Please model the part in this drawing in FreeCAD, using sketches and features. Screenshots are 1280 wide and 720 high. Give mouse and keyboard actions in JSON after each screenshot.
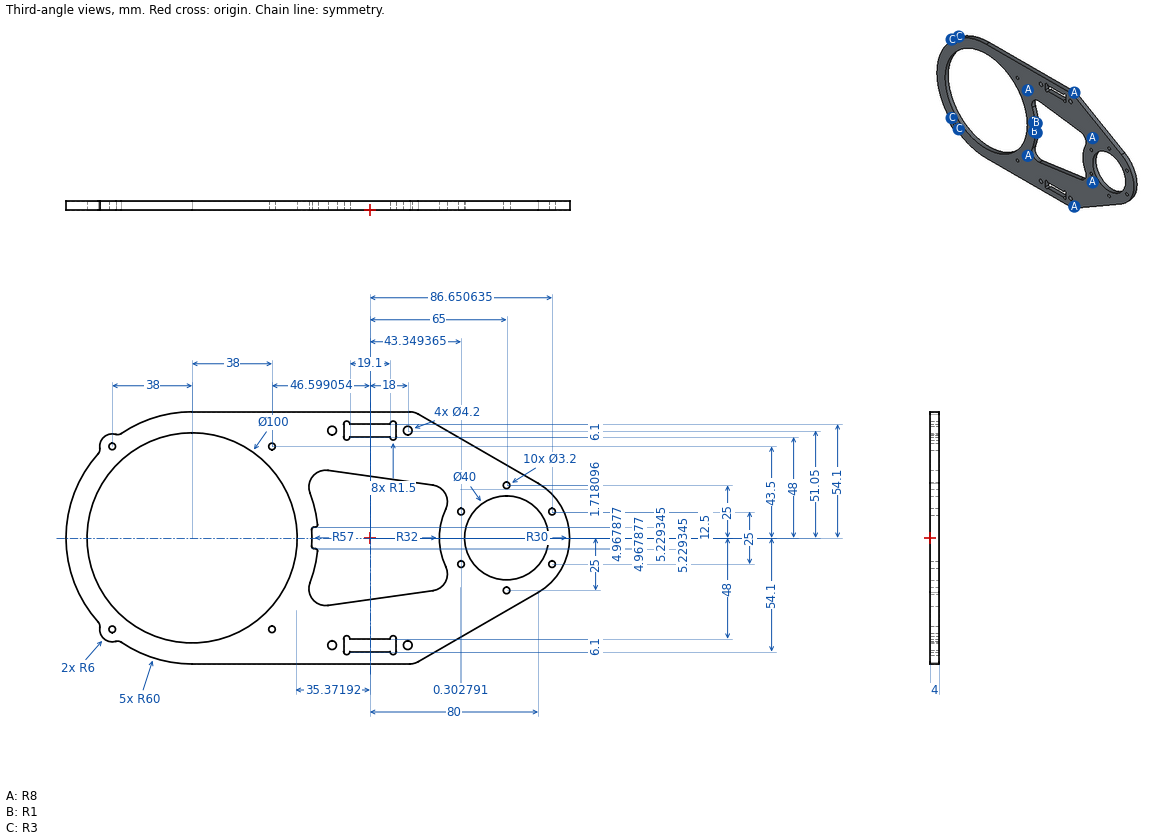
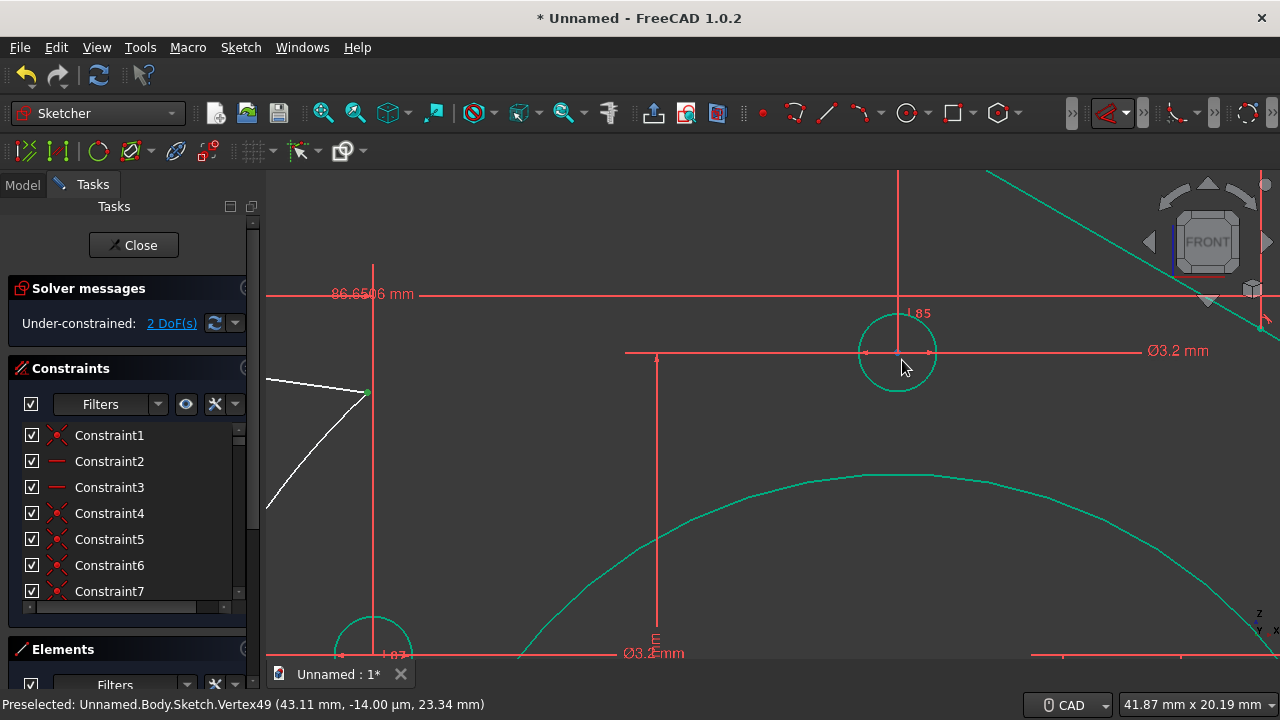
{"action": "left_click", "coordinate": [898, 353]}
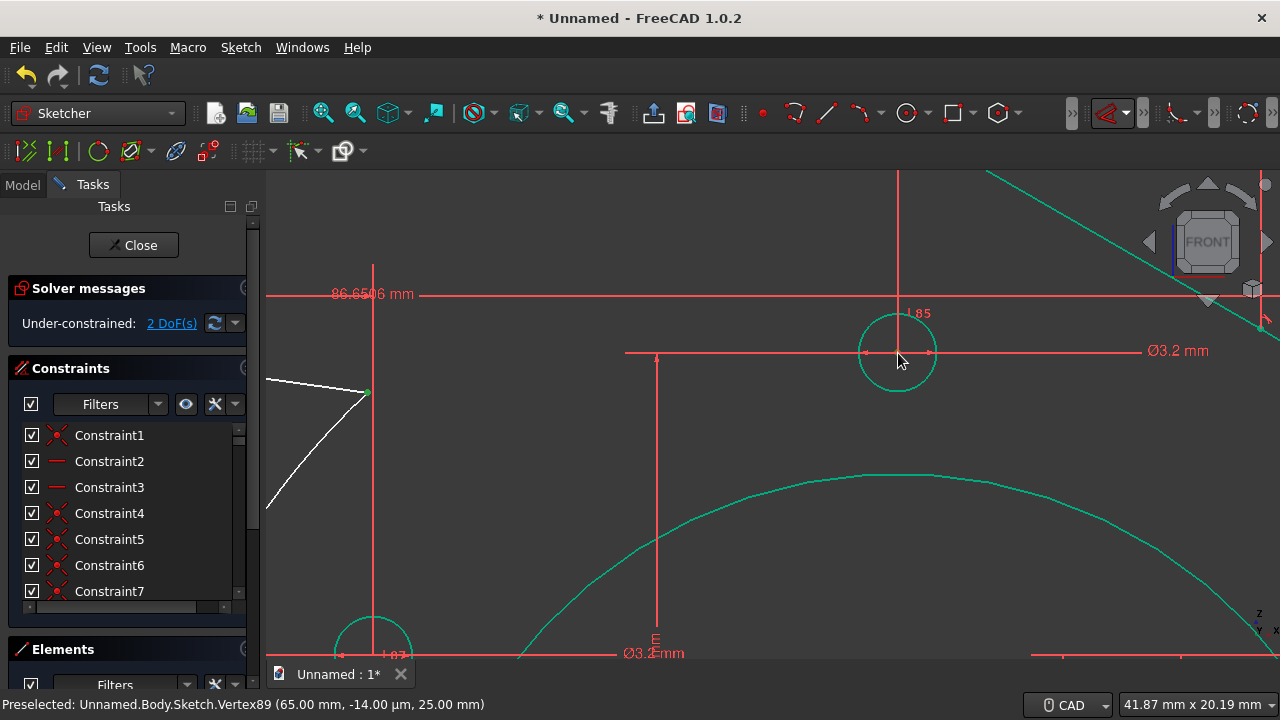
{"action": "left_click", "coordinate": [1128, 114]}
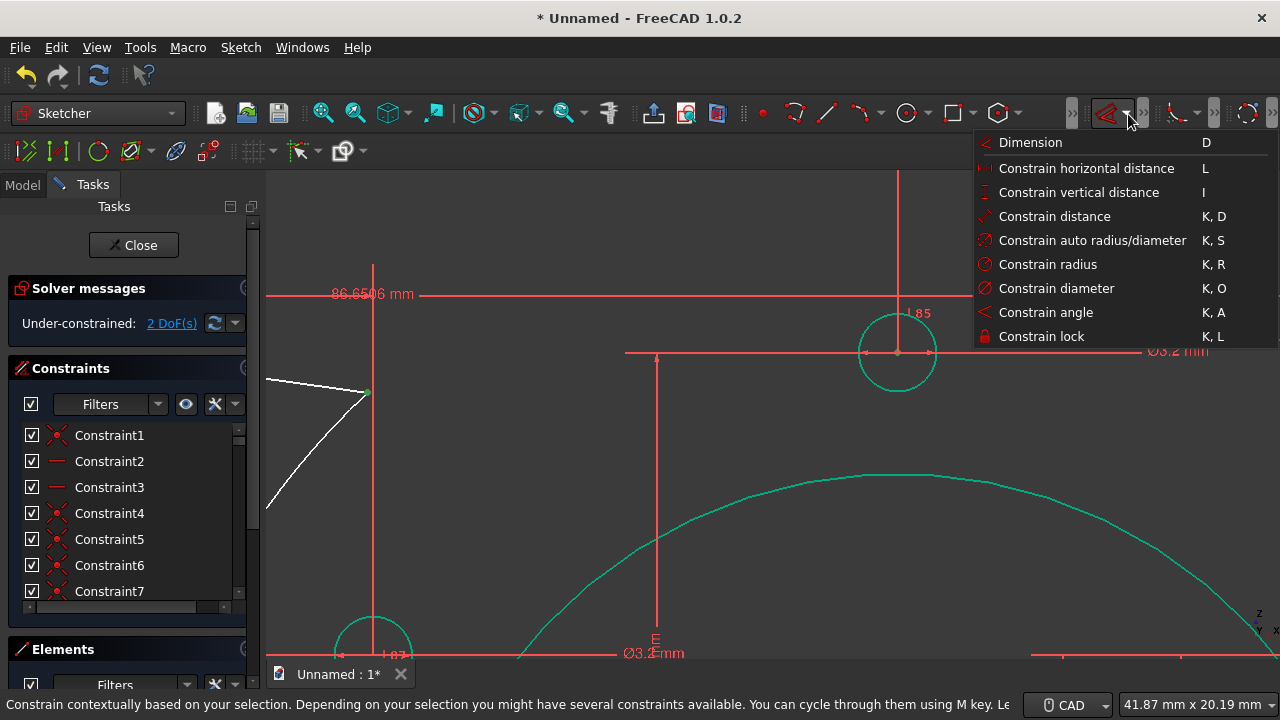
{"action": "left_click", "coordinate": [1126, 192]}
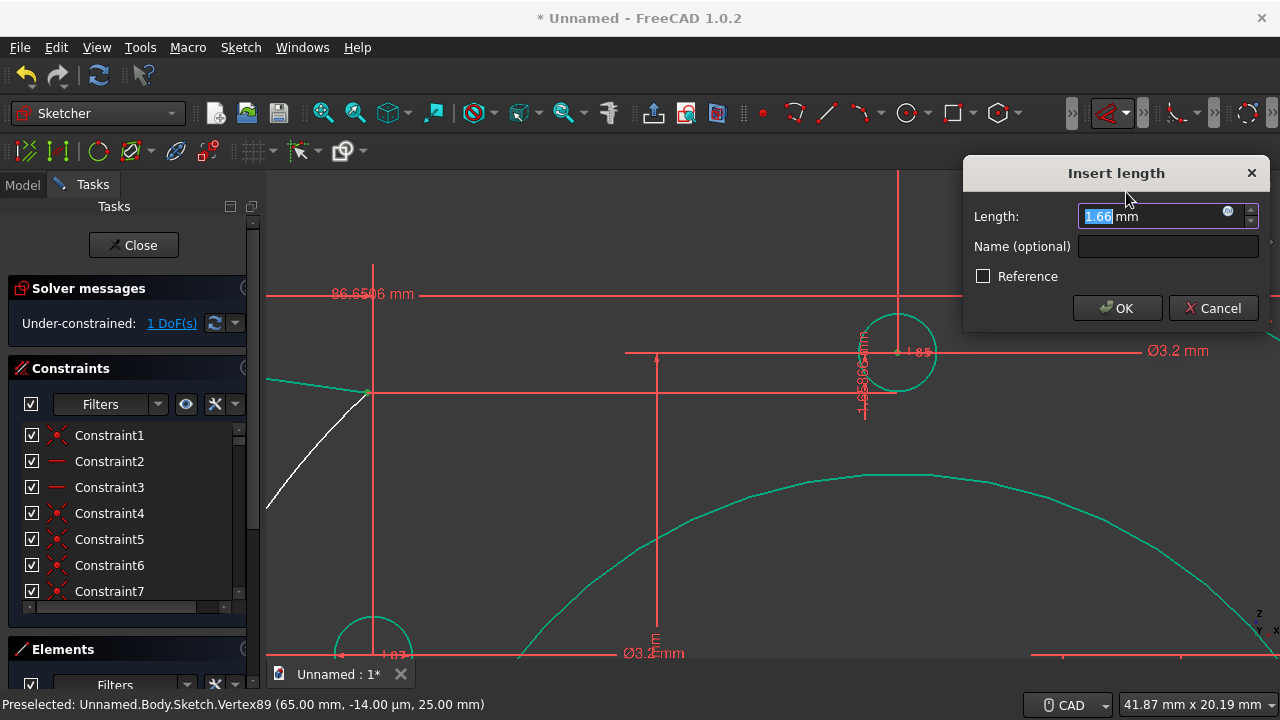
{"action": "type", "text": "1.718096"}
{"action": "key", "text": "Return"}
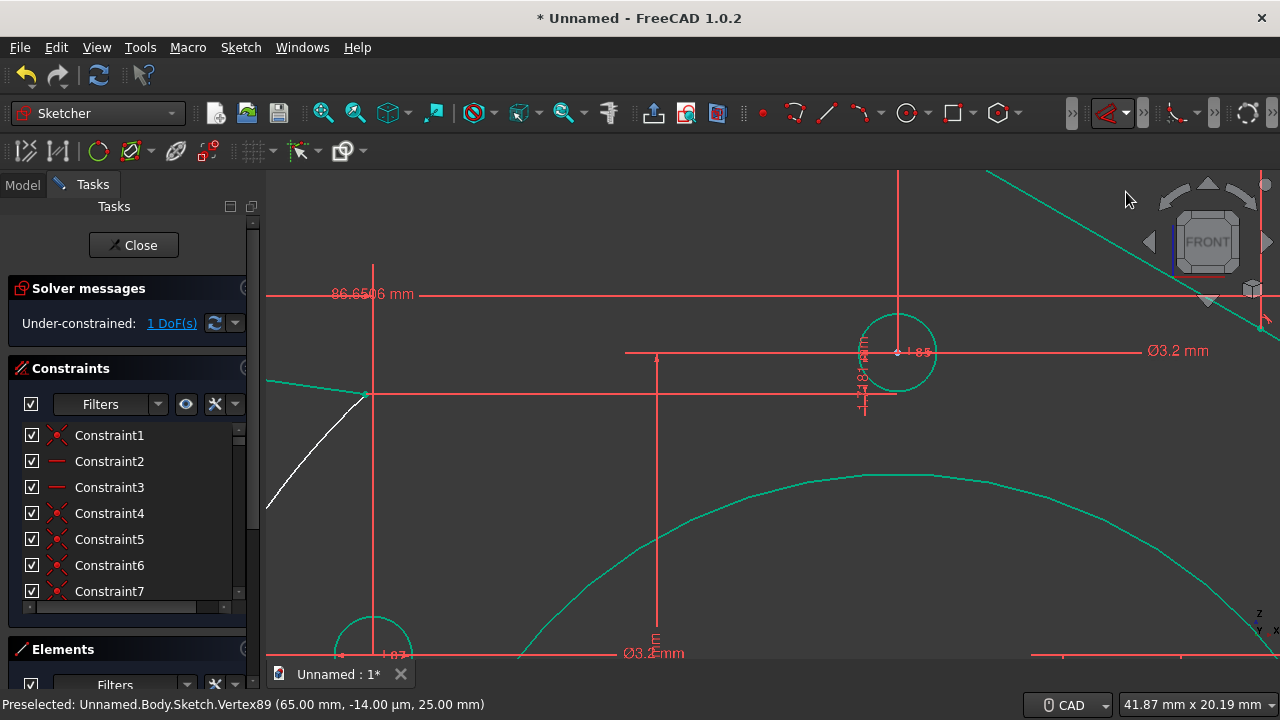
{"action": "scroll", "coordinate": [902, 360], "scroll_direction": "down", "scroll_amount": 12}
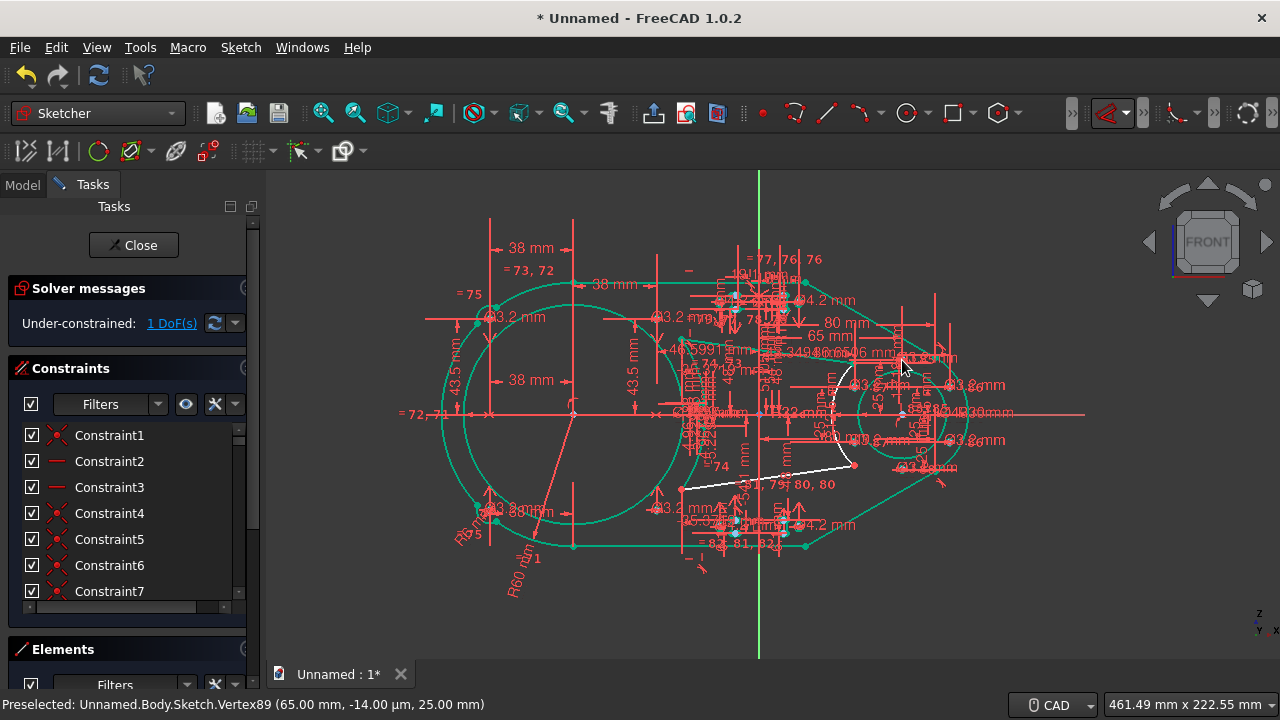
{"action": "scroll", "coordinate": [854, 466], "scroll_direction": "up", "scroll_amount": 21}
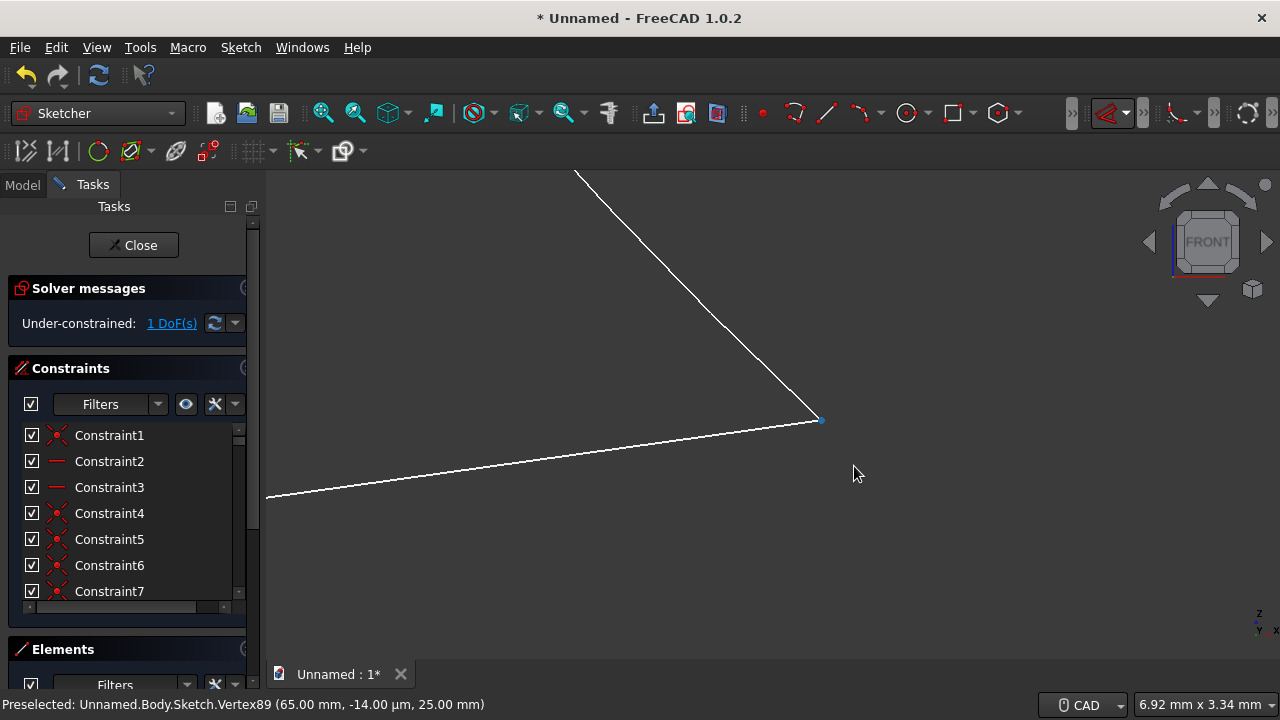
{"action": "left_click", "coordinate": [821, 420]}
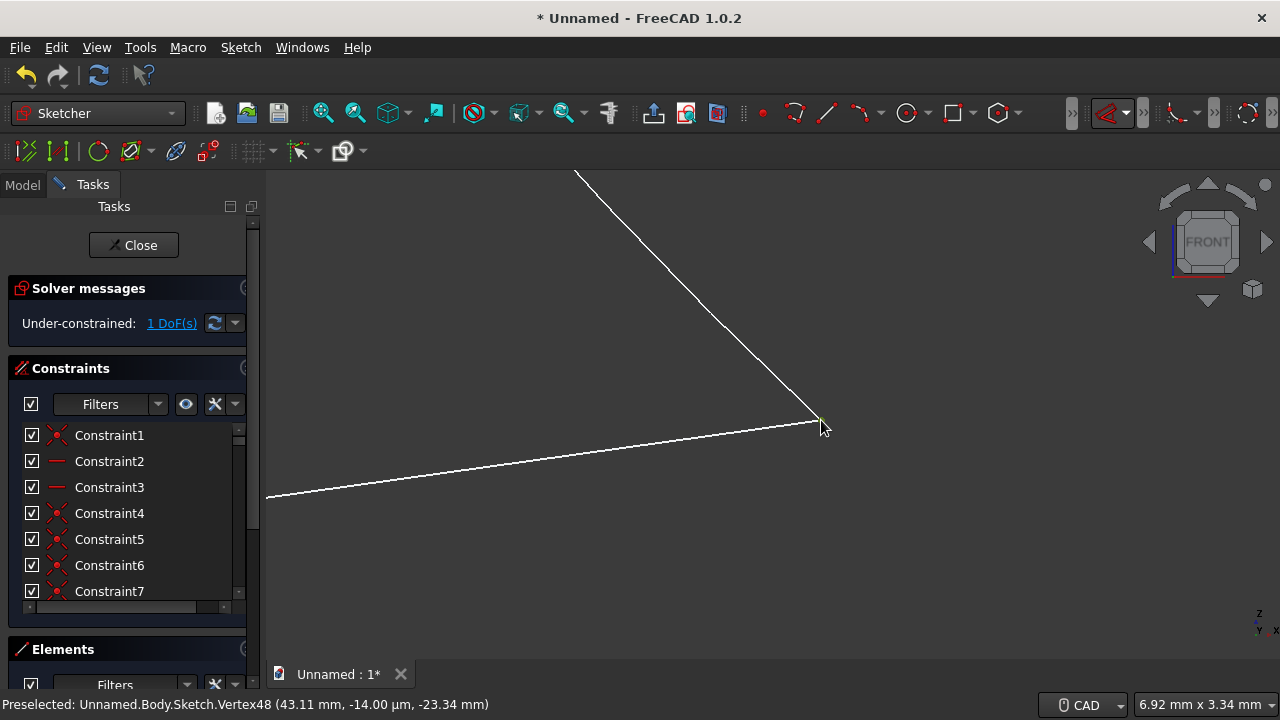
{"action": "scroll", "coordinate": [704, 414], "scroll_direction": "down", "scroll_amount": 15}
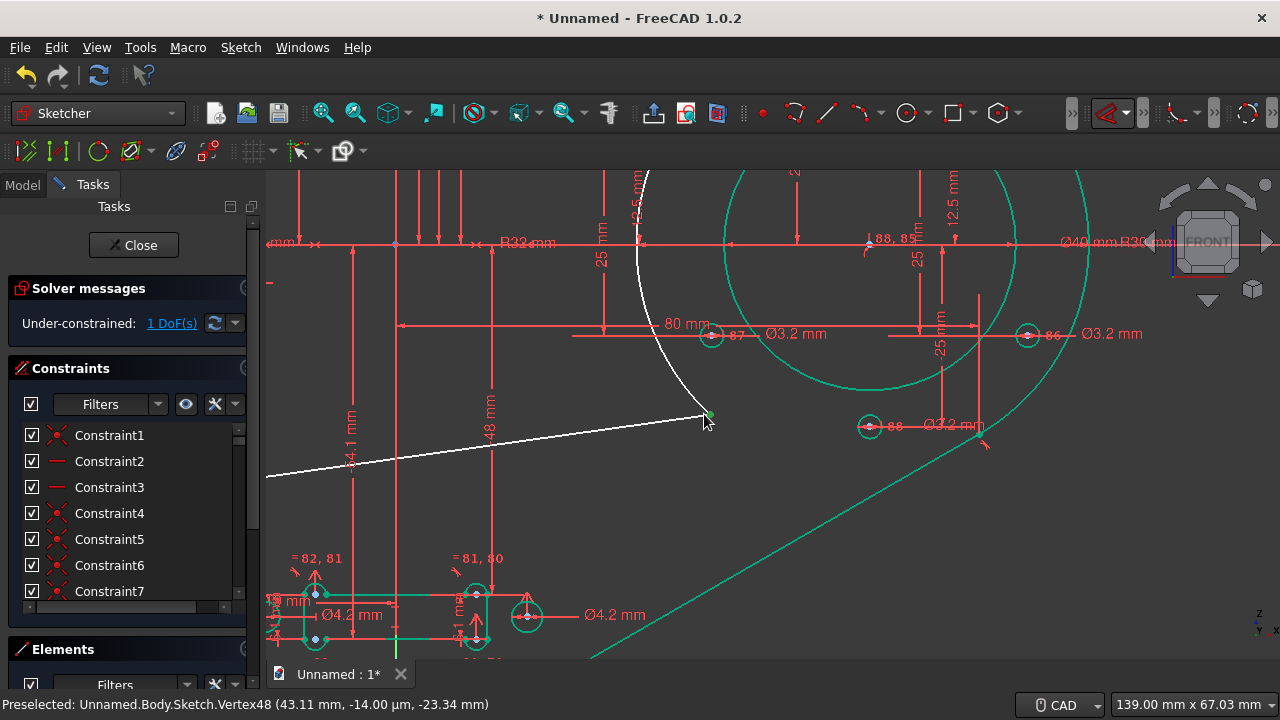
{"action": "scroll", "coordinate": [916, 488], "scroll_direction": "down", "scroll_amount": 6}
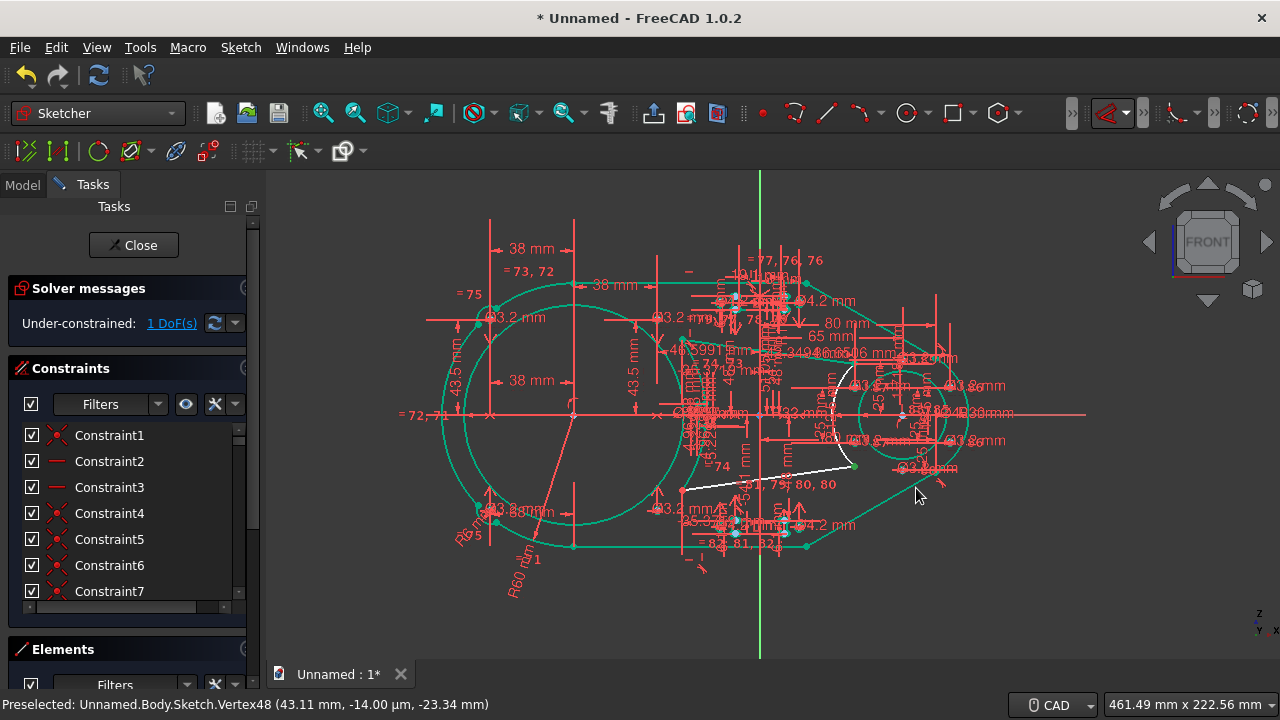
{"action": "scroll", "coordinate": [855, 388], "scroll_direction": "up", "scroll_amount": 21}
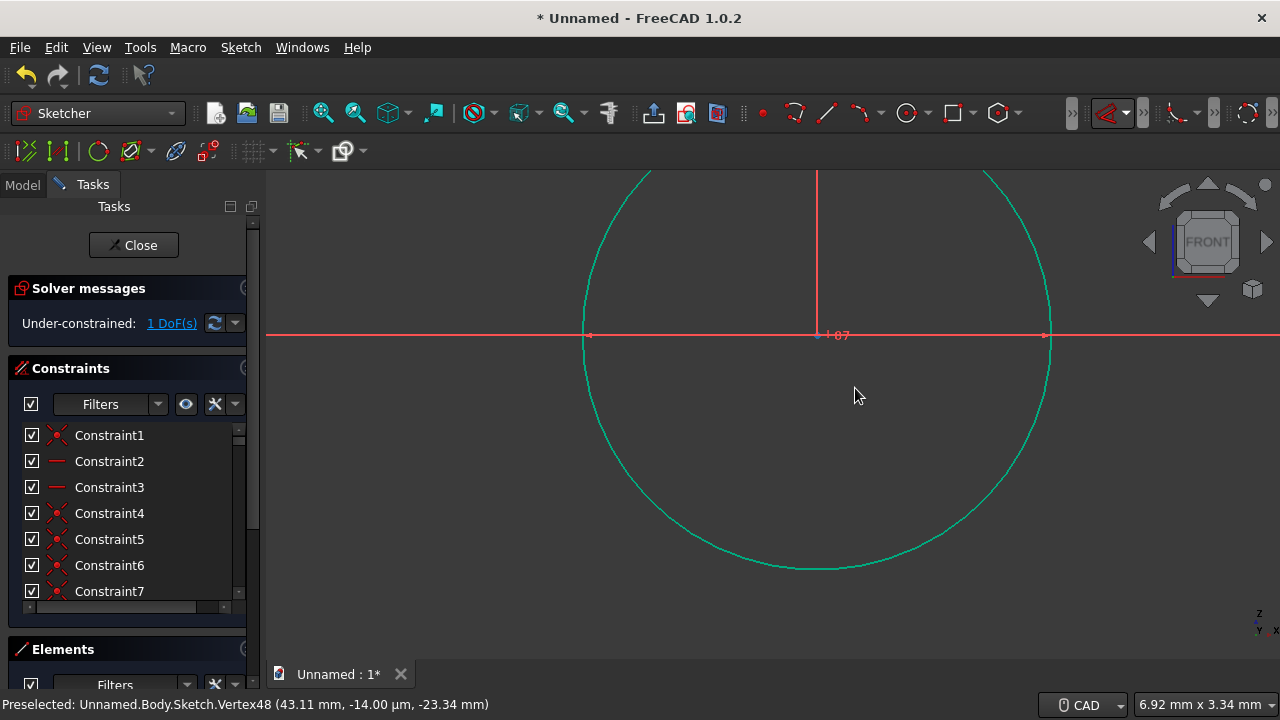
{"action": "left_click", "coordinate": [817, 335]}